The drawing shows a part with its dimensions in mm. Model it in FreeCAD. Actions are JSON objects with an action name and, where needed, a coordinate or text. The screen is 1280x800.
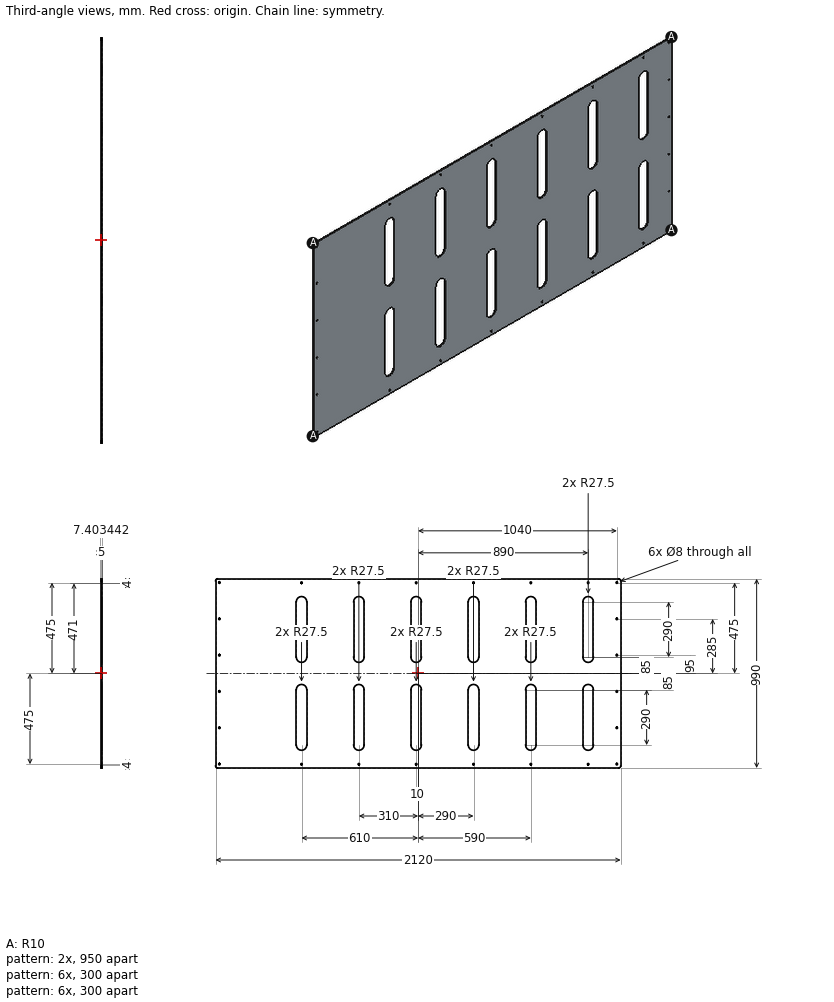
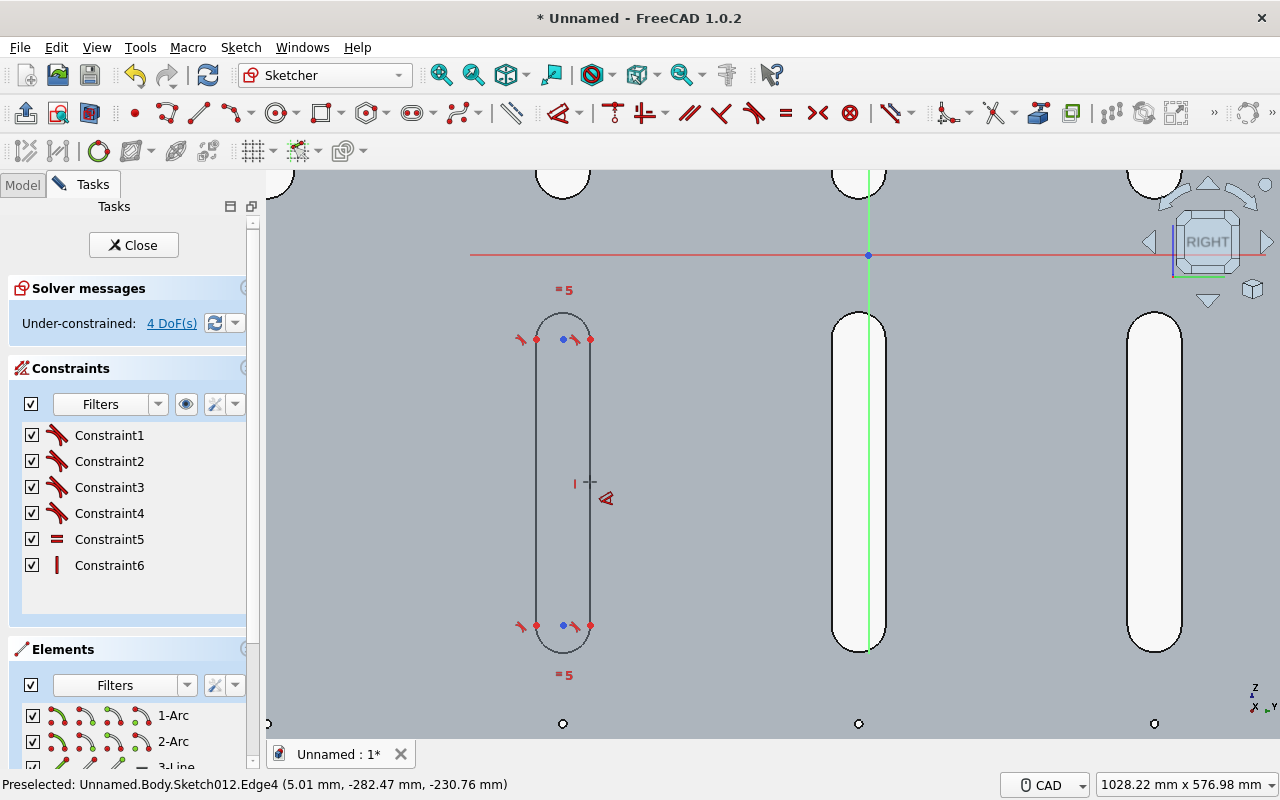
{"action": "scroll", "coordinate": [547, 648], "scroll_direction": "up", "scroll_amount": 2}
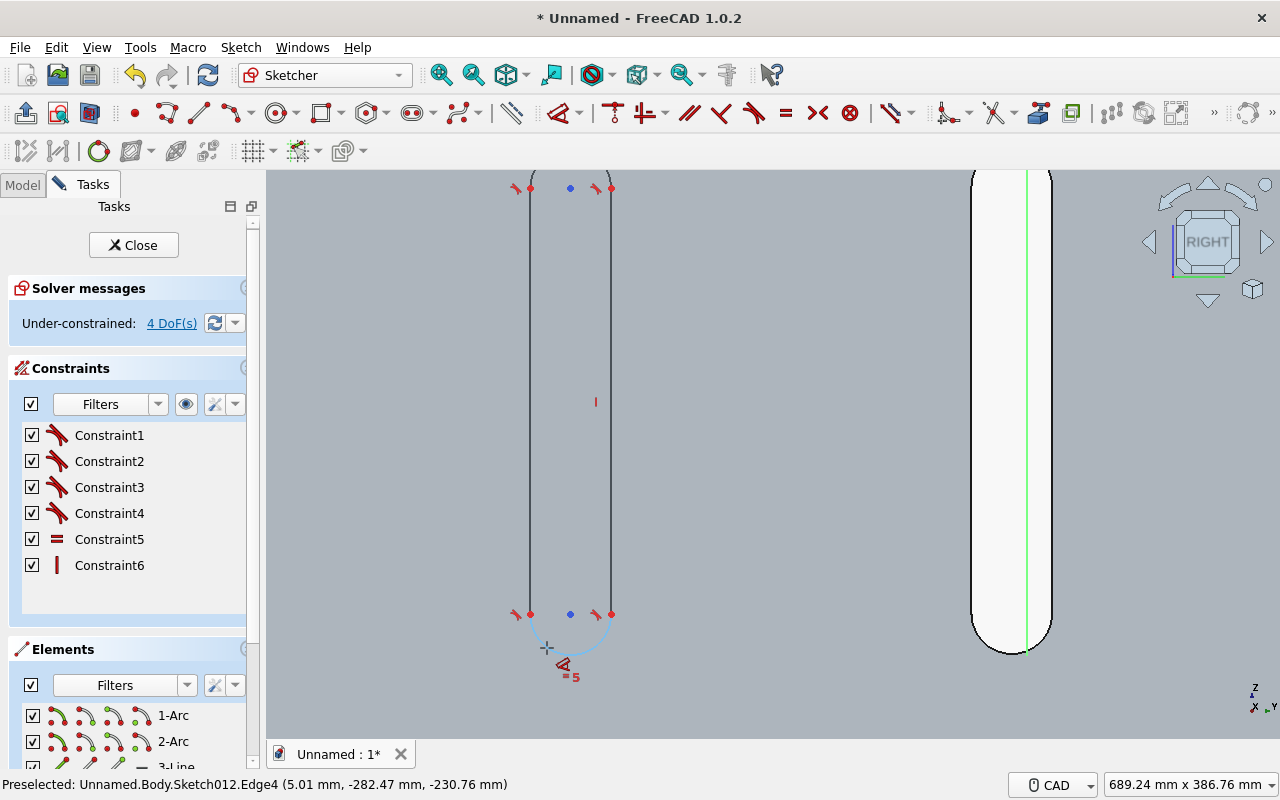
{"action": "left_click", "coordinate": [547, 647]}
{"action": "left_click", "coordinate": [528, 673]}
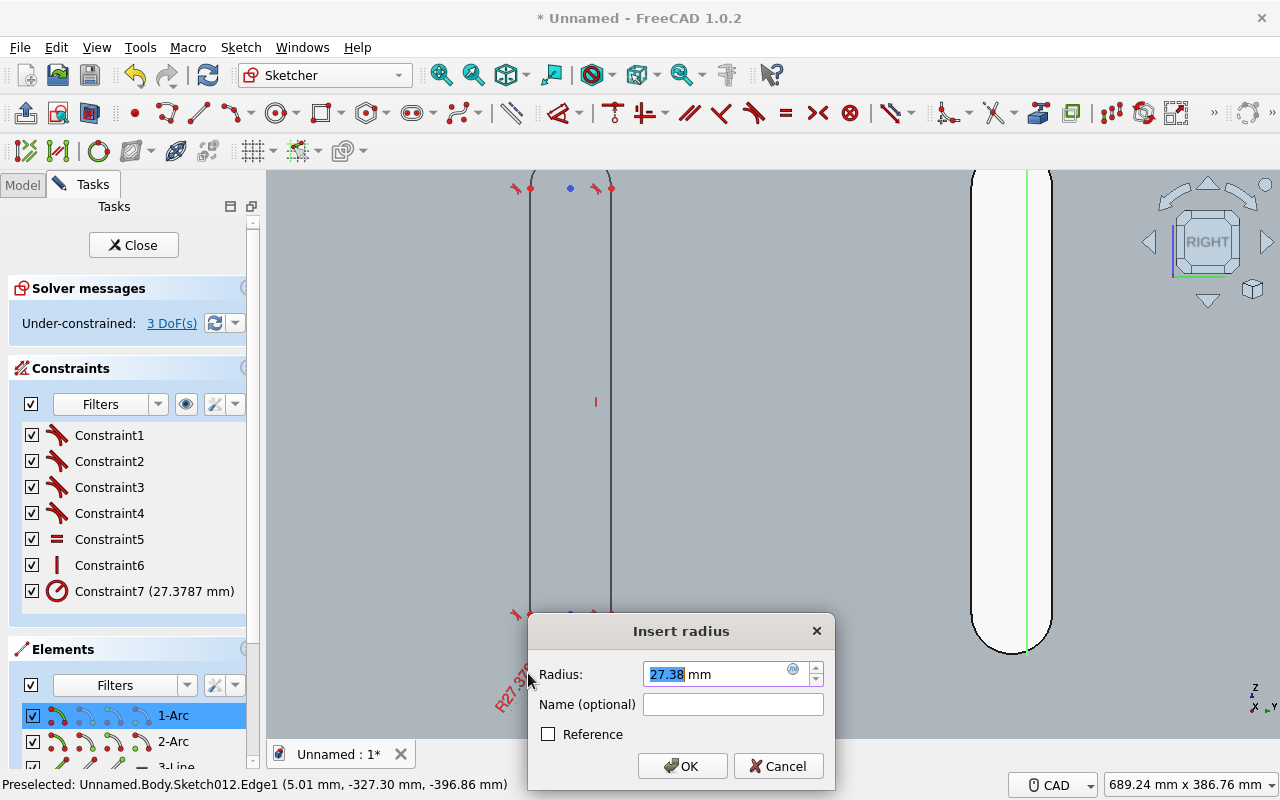
{"action": "type", "text": "27.5"}
{"action": "key", "text": "Return"}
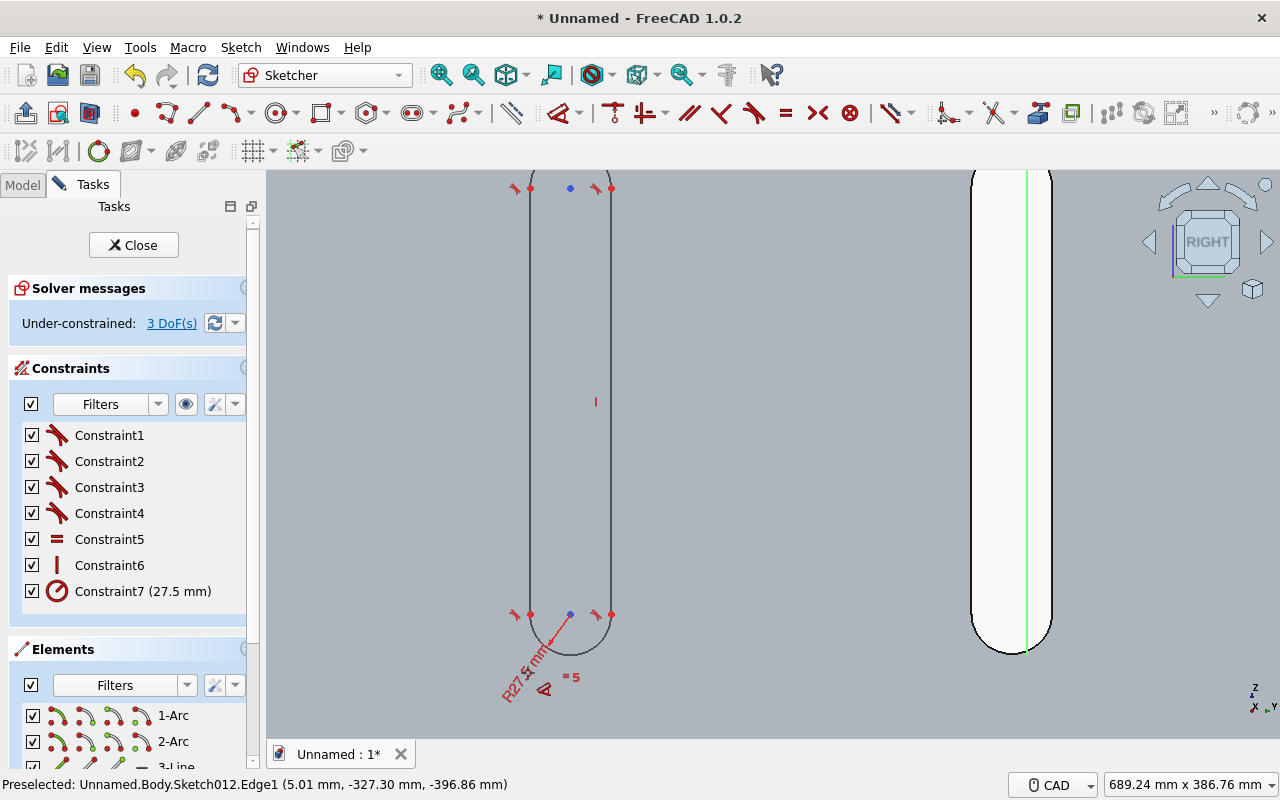
{"action": "left_click", "coordinate": [530, 487]}
{"action": "left_click", "coordinate": [496, 406]}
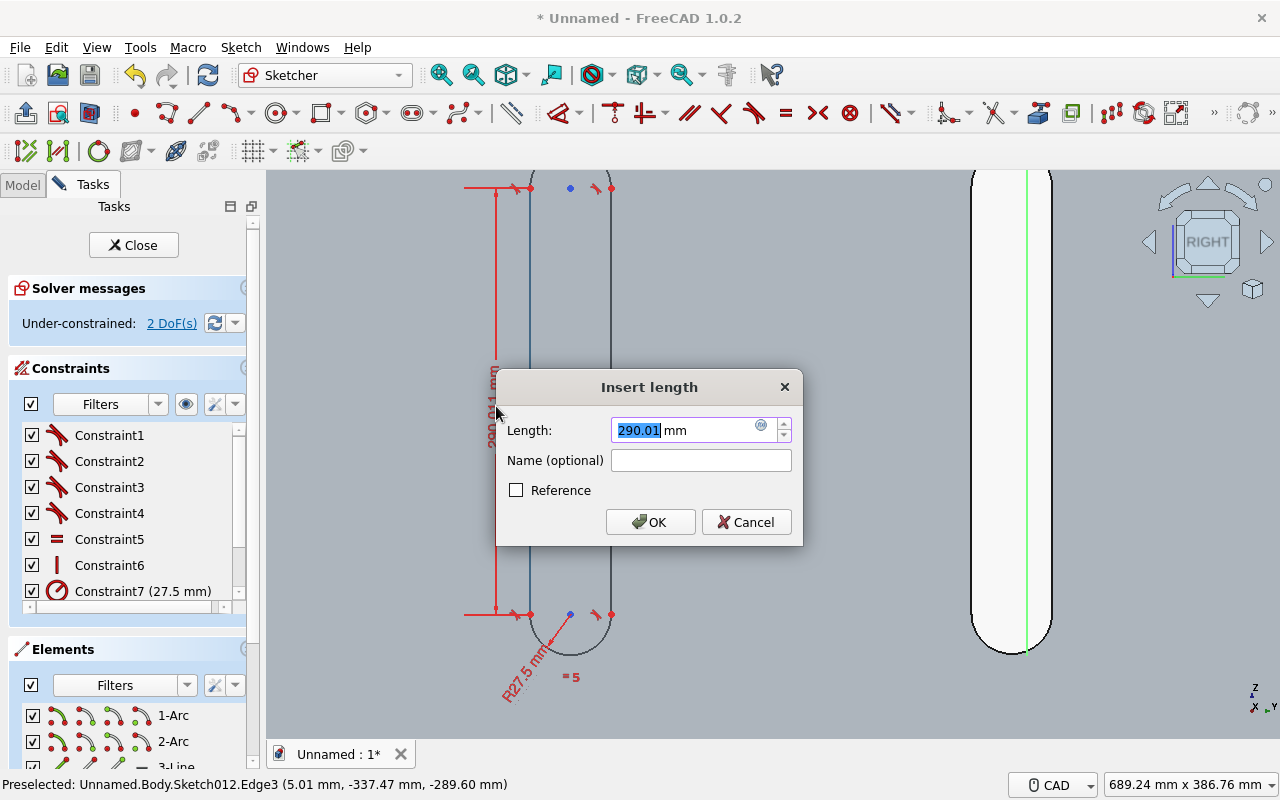
{"action": "type", "text": "290"}
{"action": "key", "text": "Return"}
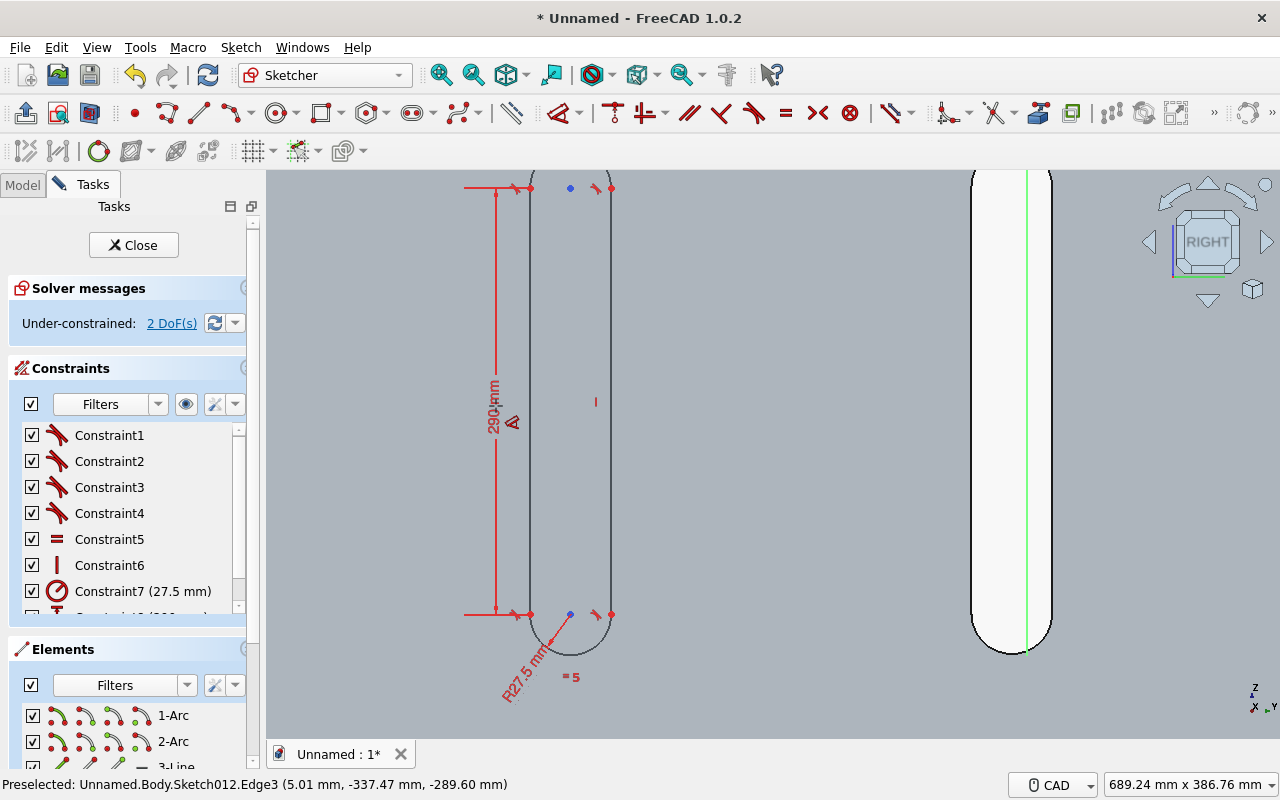
{"action": "scroll", "coordinate": [554, 651], "scroll_direction": "down", "scroll_amount": 2}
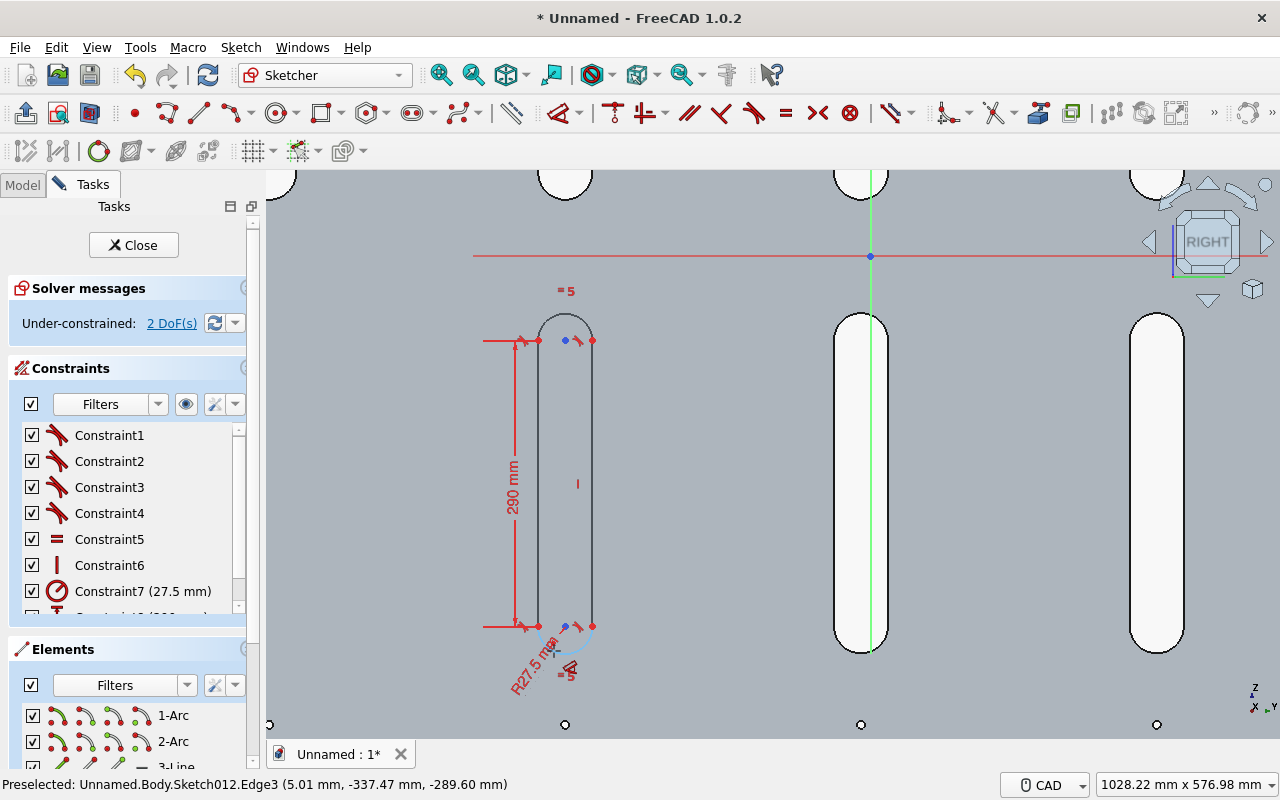
{"action": "left_click", "coordinate": [592, 341]}
{"action": "left_click", "coordinate": [905, 299]}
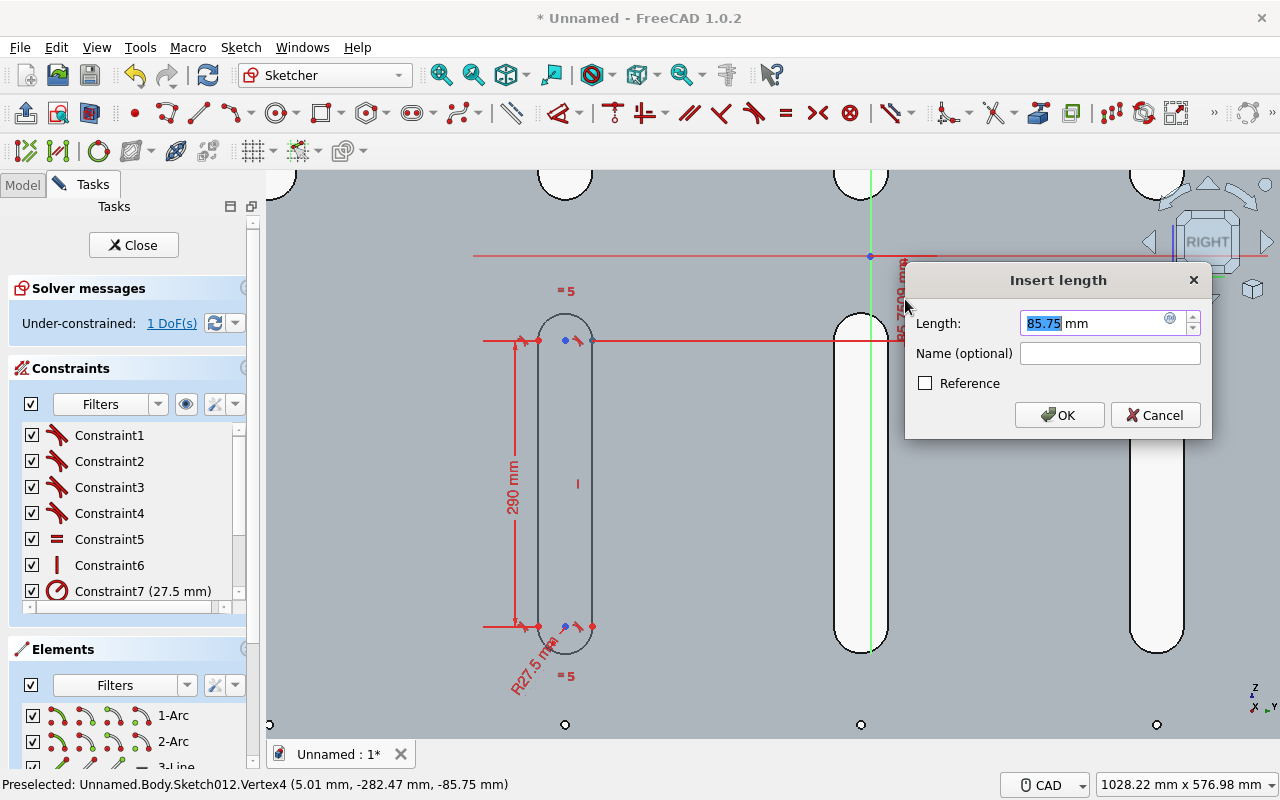
{"action": "type", "text": "85"}
{"action": "key", "text": "Return"}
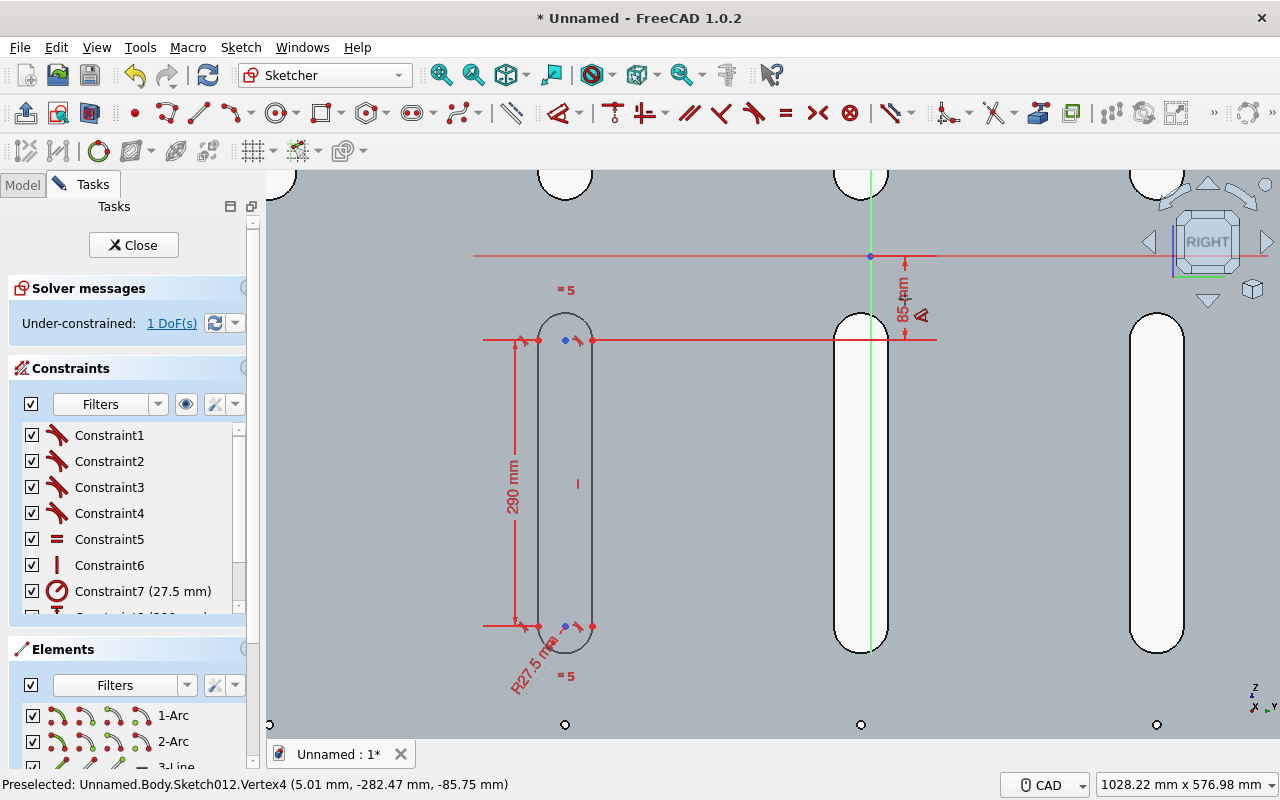
{"action": "left_click", "coordinate": [565, 626]}
{"action": "left_click", "coordinate": [718, 222]}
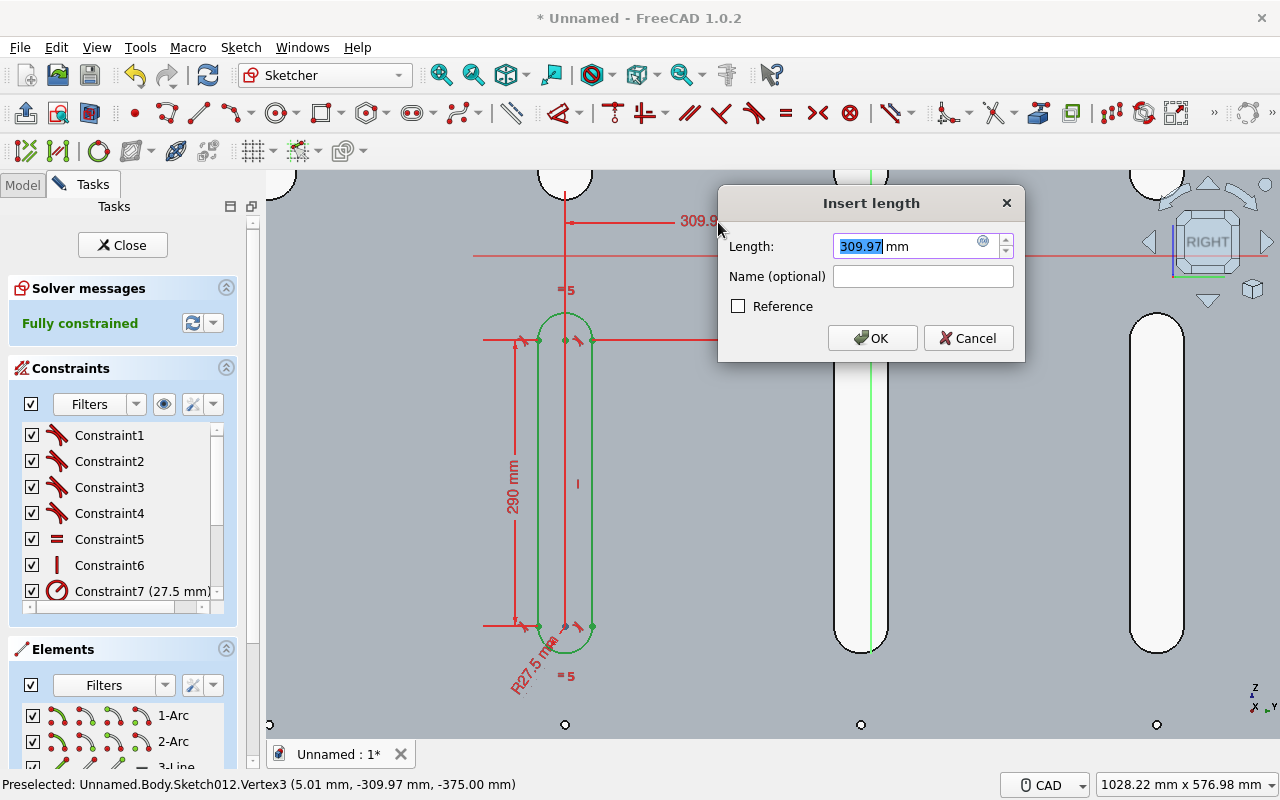
{"action": "type", "text": "310"}
{"action": "key", "text": "Return"}
{"action": "key", "text": "Escape"}